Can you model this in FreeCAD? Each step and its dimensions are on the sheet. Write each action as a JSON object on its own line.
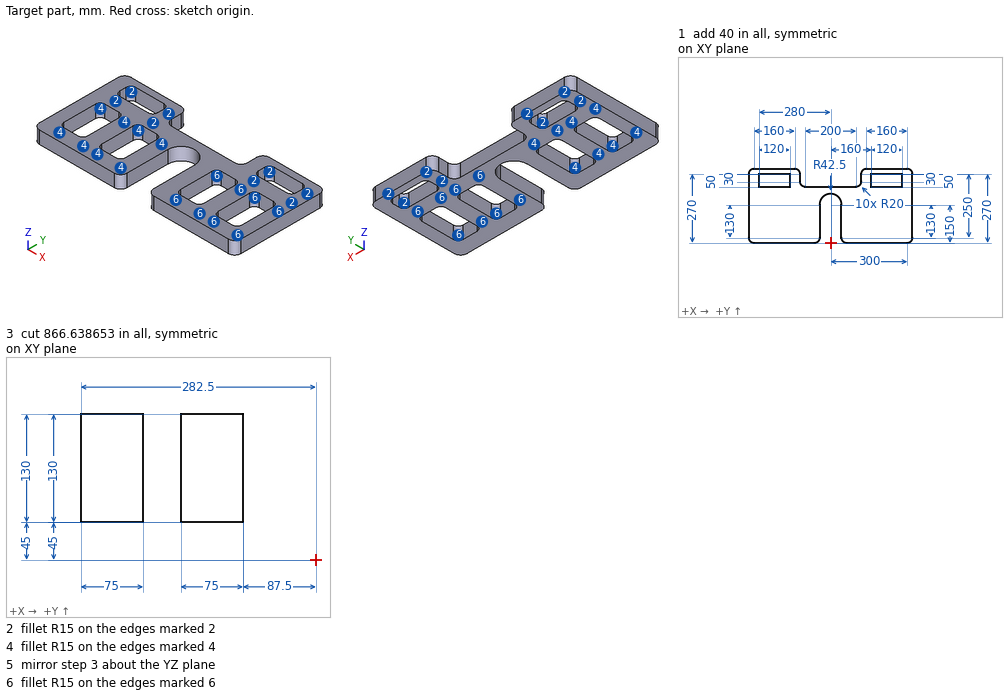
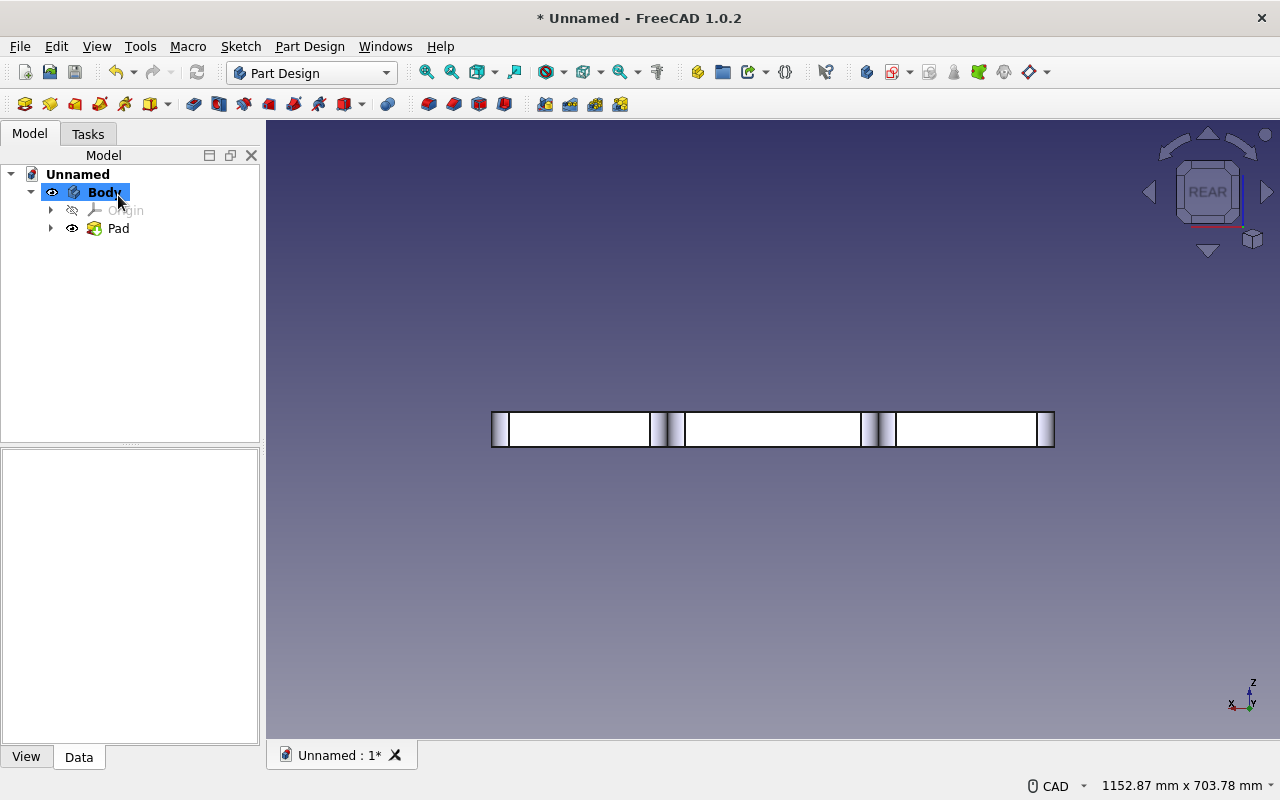
{"action": "key", "text": "6"}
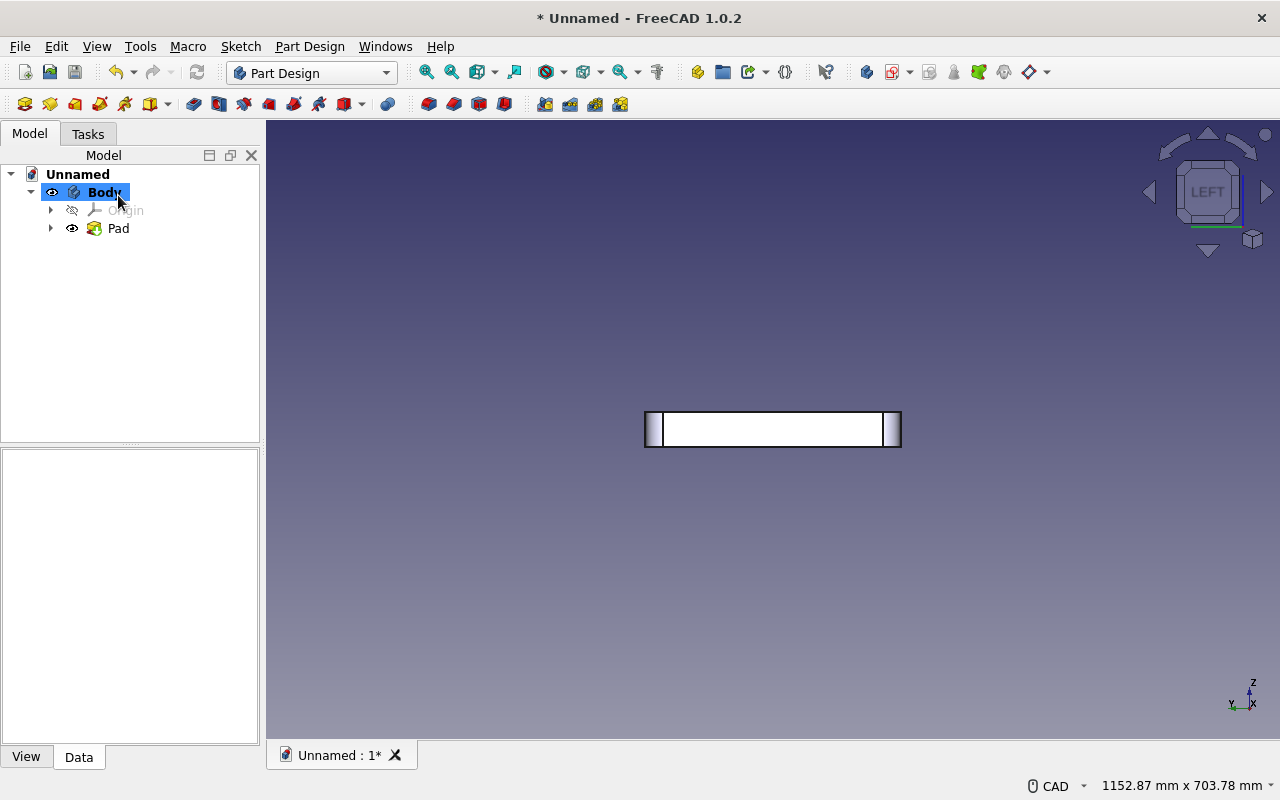
{"action": "left_click", "coordinate": [427, 72]}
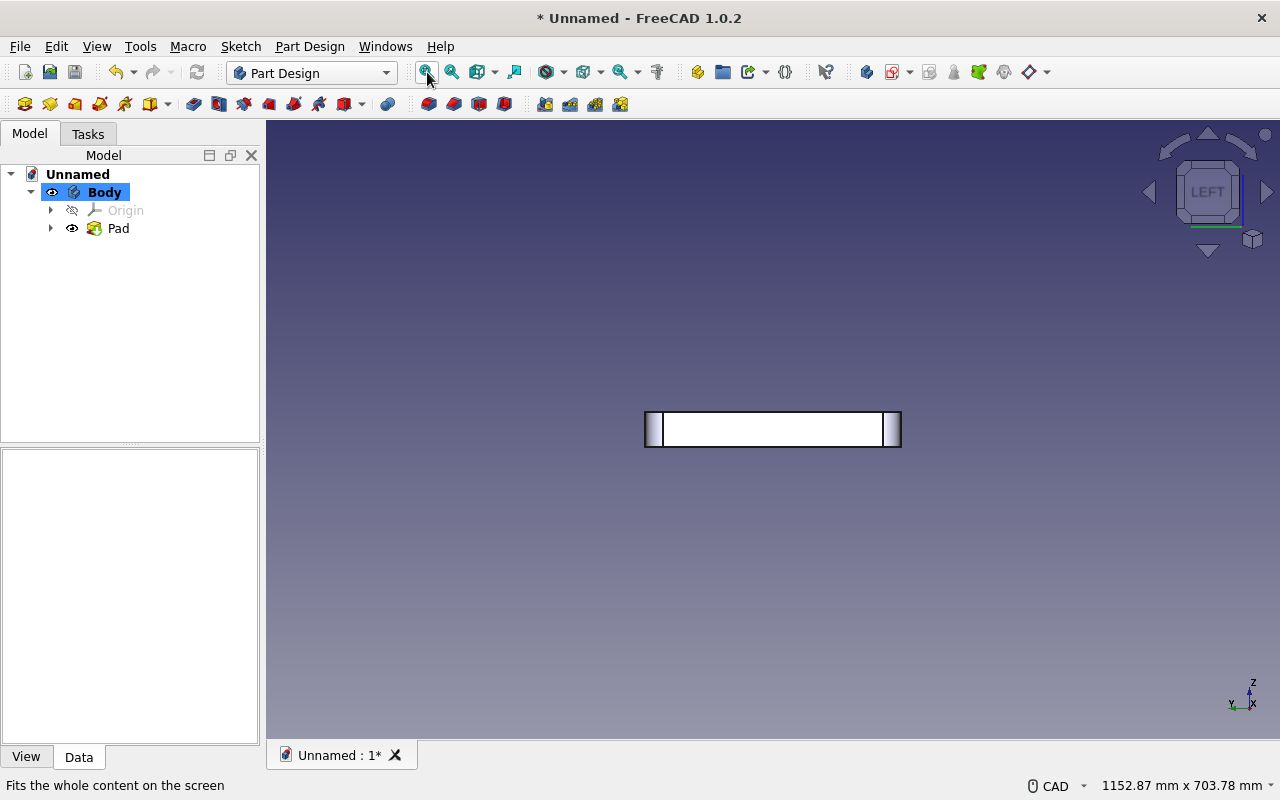
{"action": "key", "text": "v 3"}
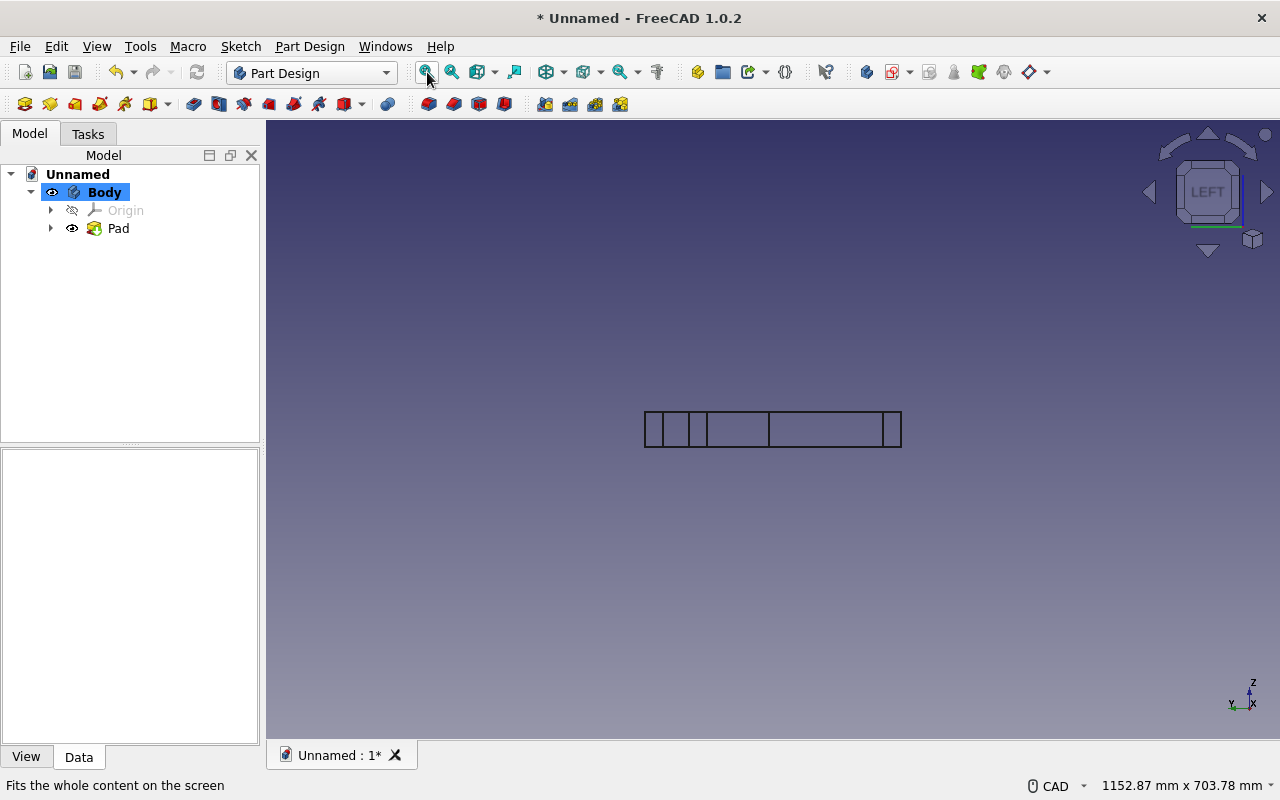
{"action": "key", "text": "0"}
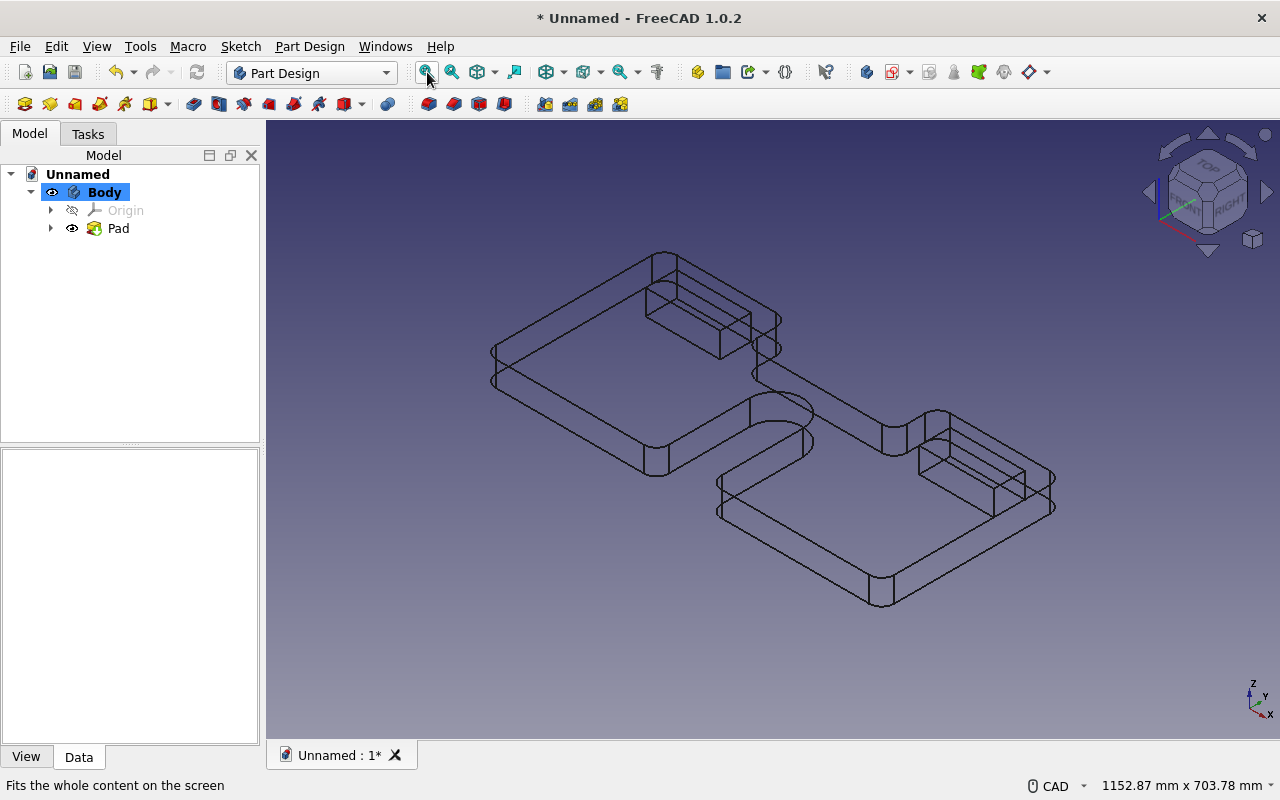
{"action": "left_click", "coordinate": [720, 344]}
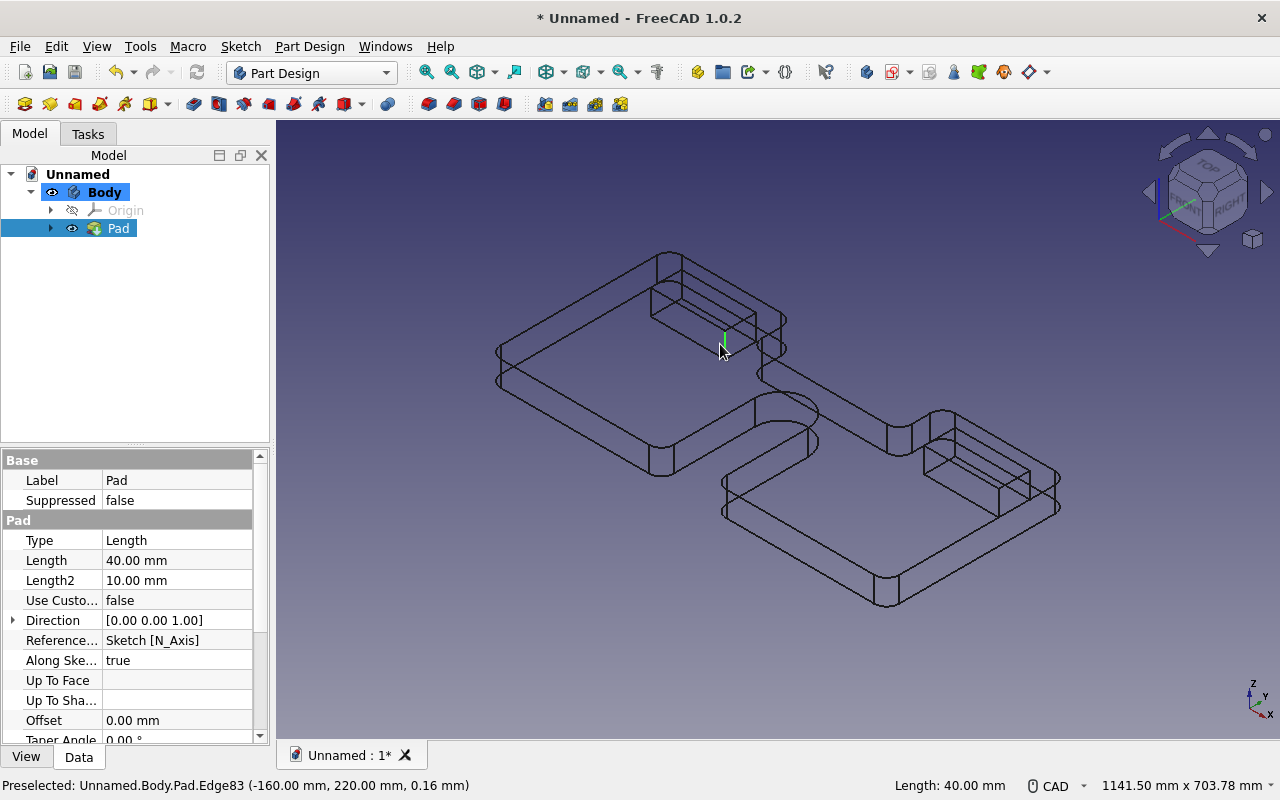
{"action": "left_click", "coordinate": [756, 326], "text": "ctrl"}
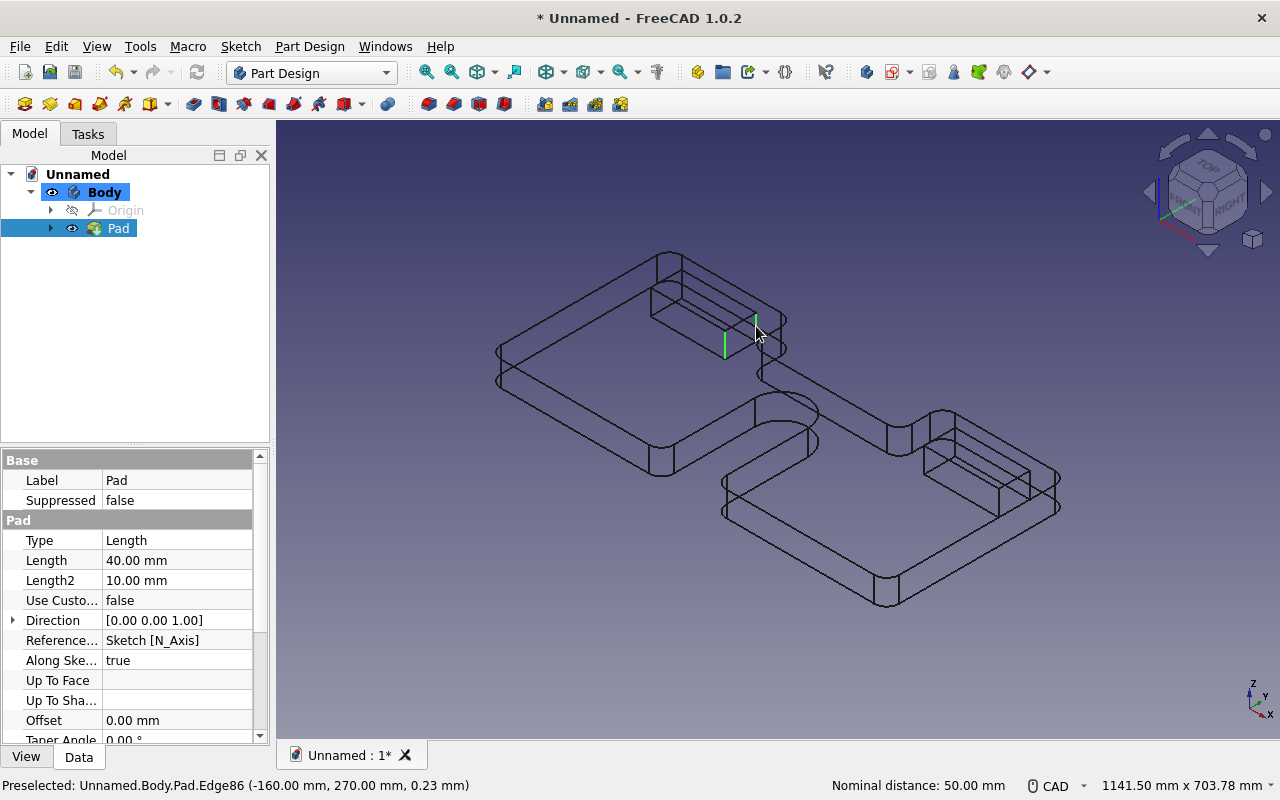
{"action": "left_click", "coordinate": [682, 283], "text": "ctrl"}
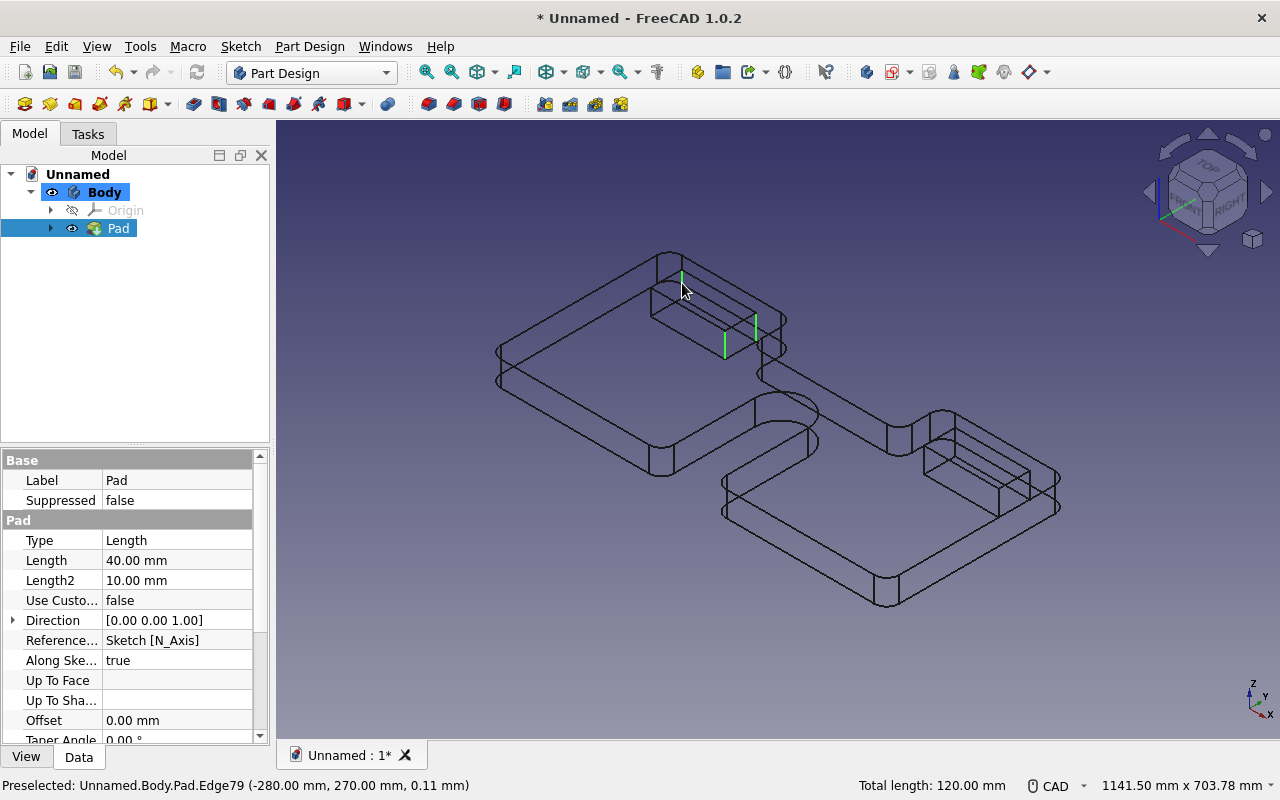
{"action": "left_click", "coordinate": [651, 301], "text": "ctrl"}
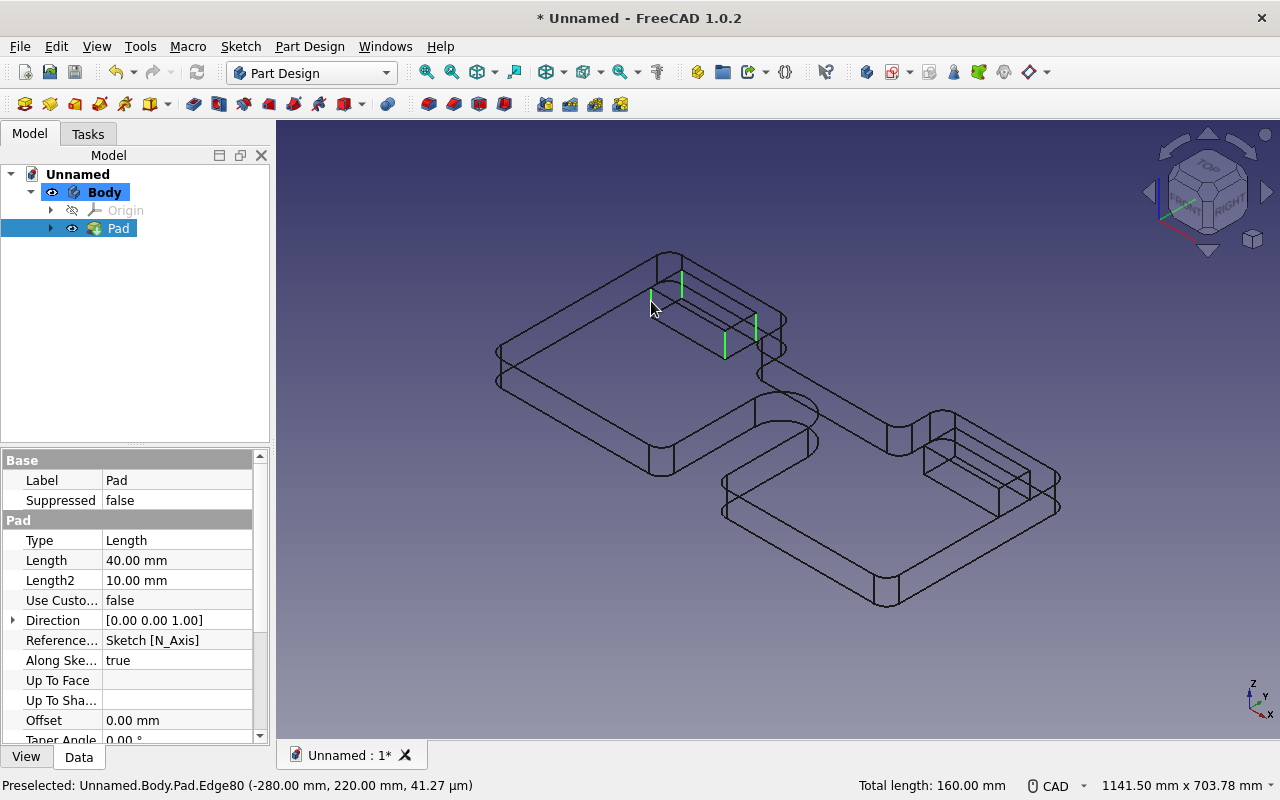
{"action": "left_click", "coordinate": [999, 502], "text": "ctrl"}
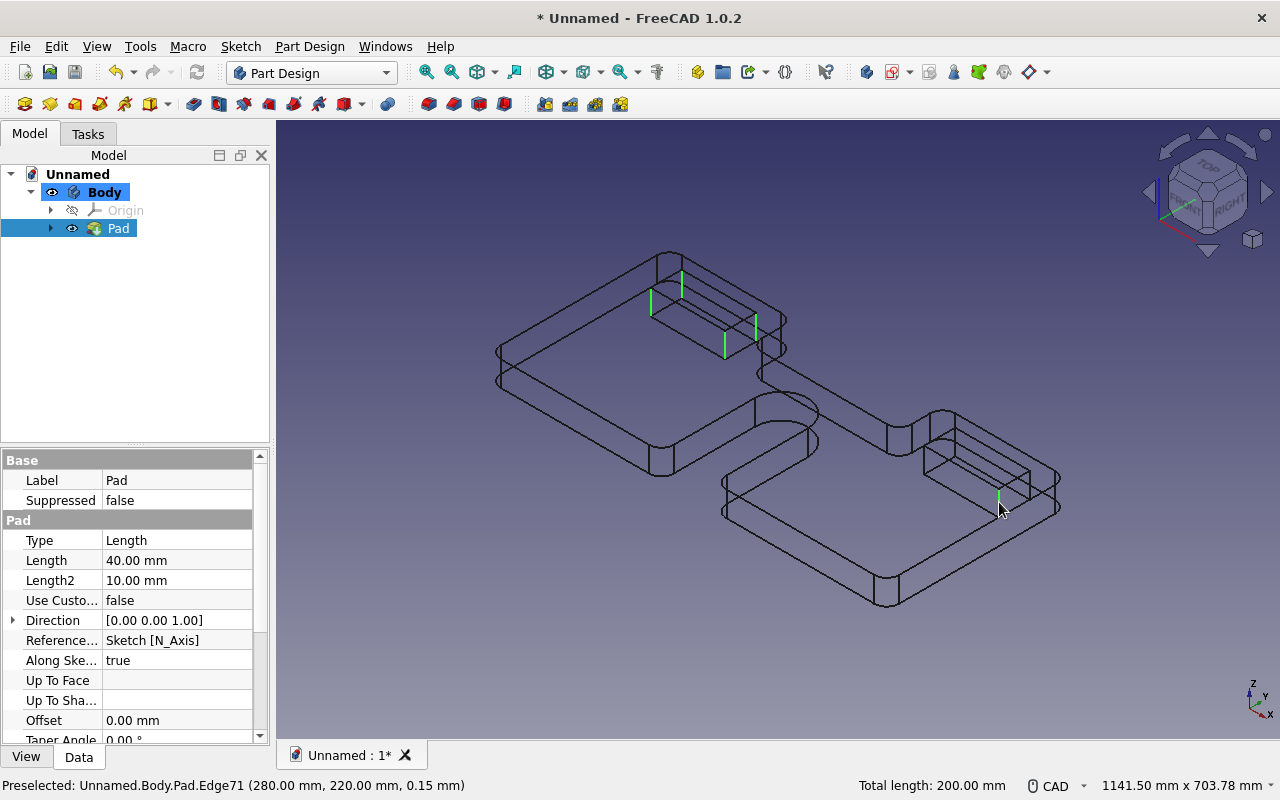
{"action": "left_click", "coordinate": [1030, 484], "text": "ctrl"}